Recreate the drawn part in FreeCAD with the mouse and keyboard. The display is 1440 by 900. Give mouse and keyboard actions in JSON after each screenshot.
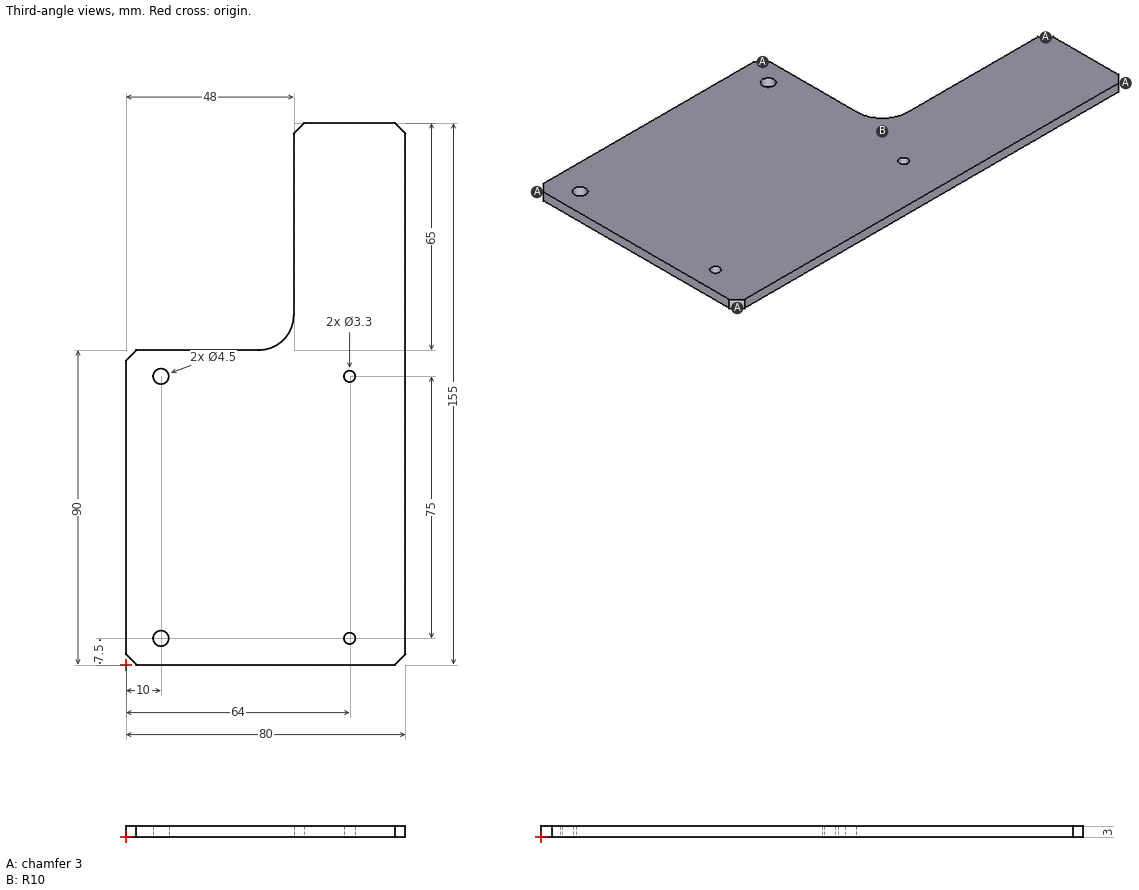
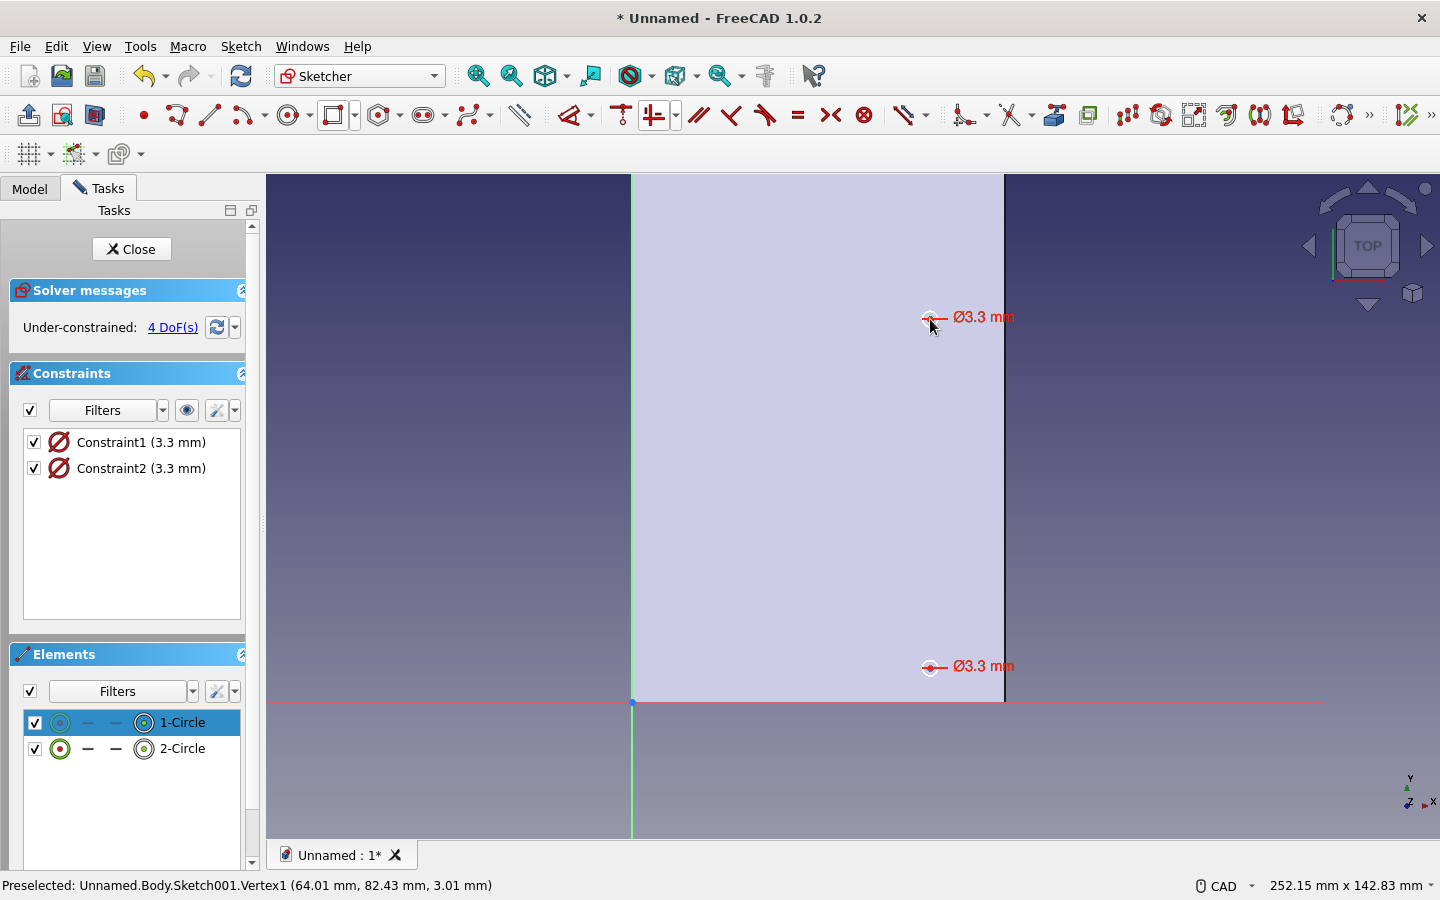
{"action": "left_click", "coordinate": [930, 668]}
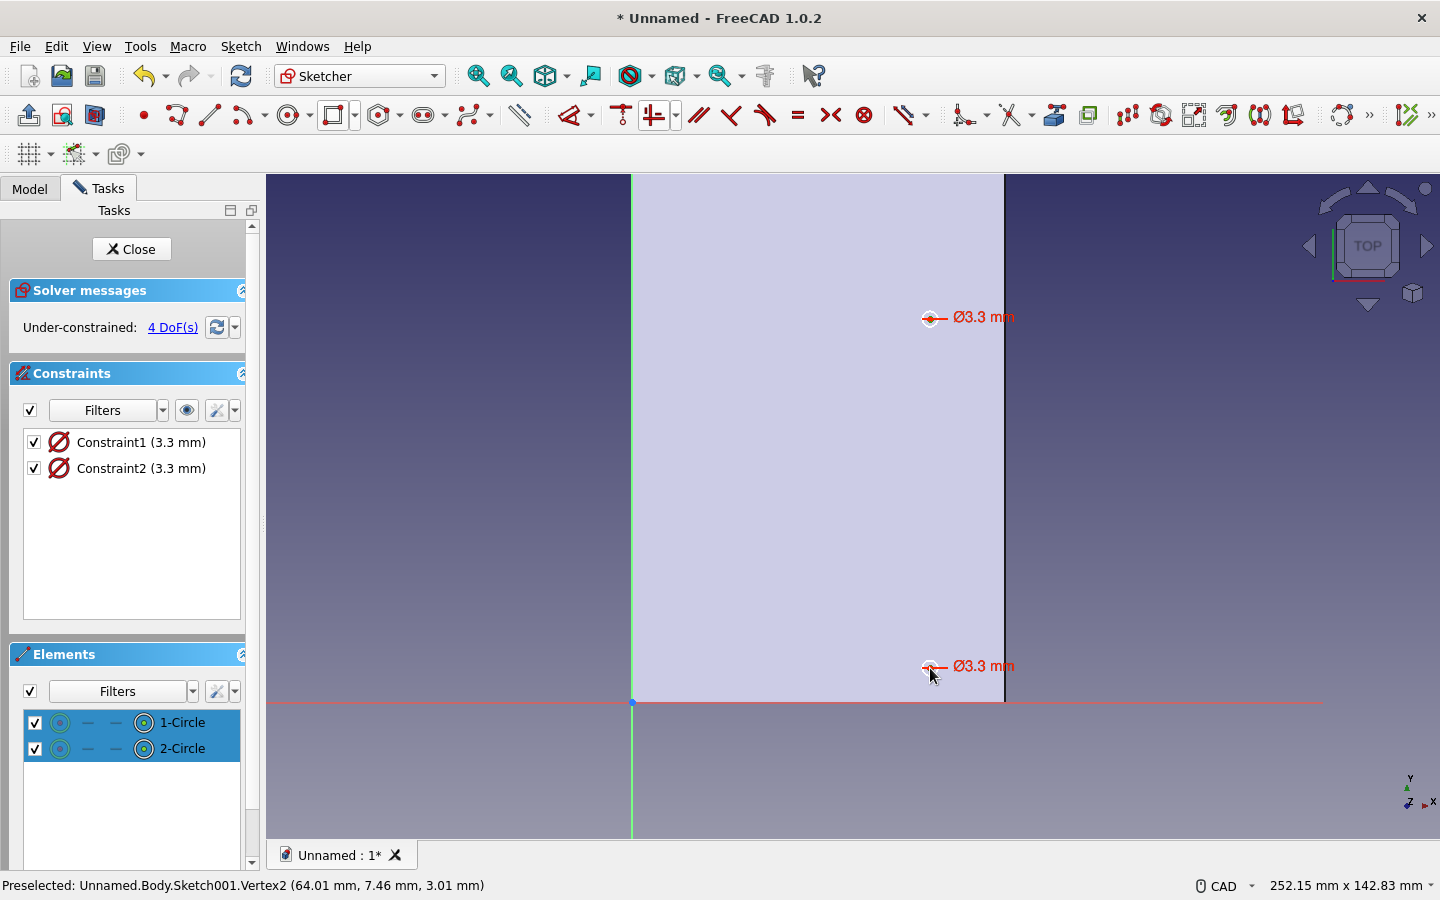
{"action": "key", "text": "v"}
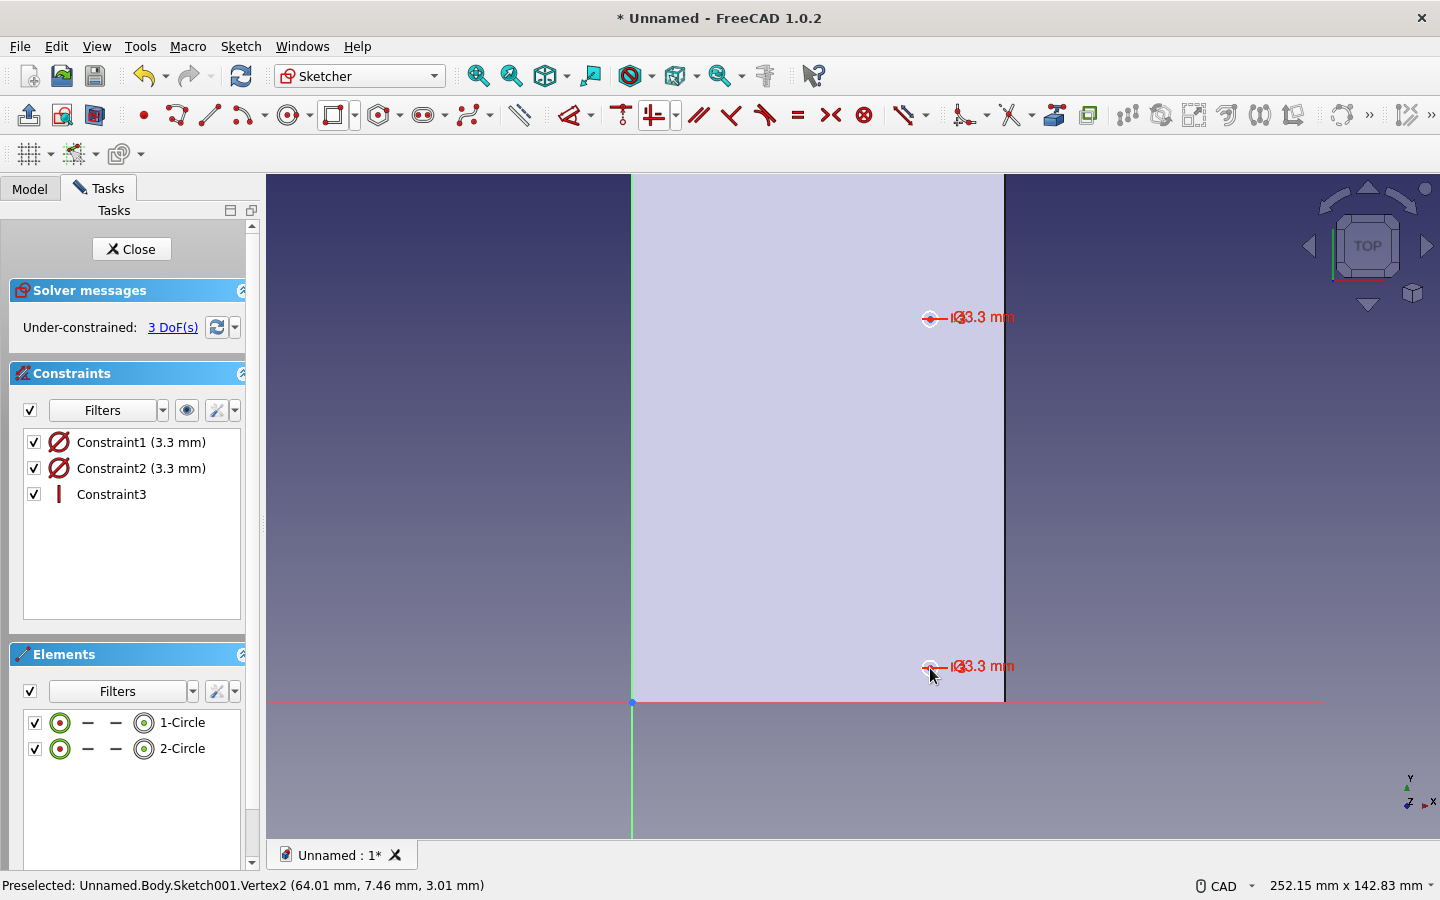
{"action": "key", "text": "d"}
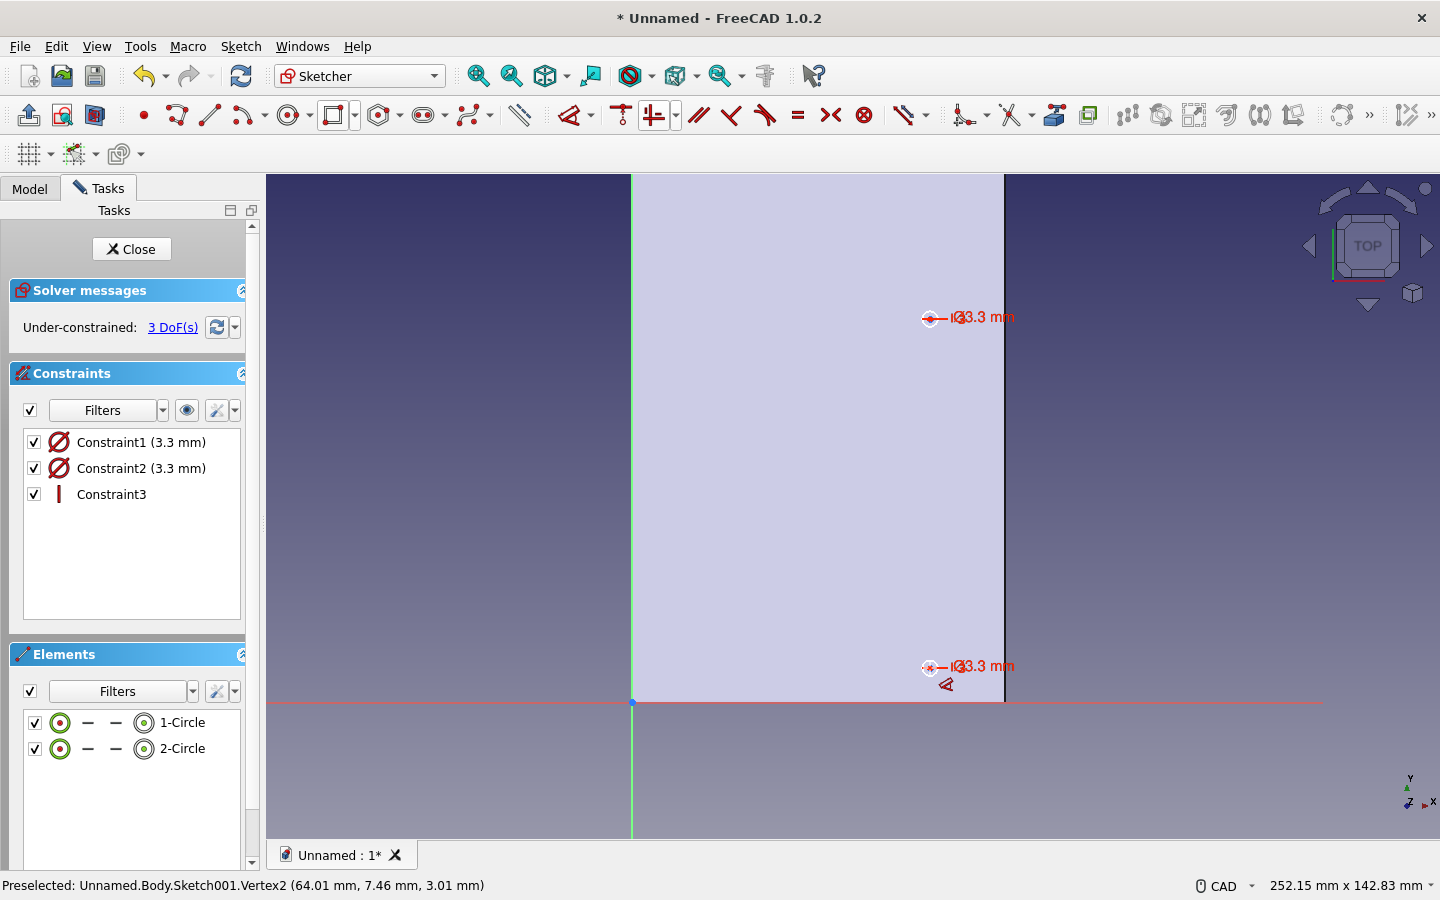
{"action": "left_click", "coordinate": [930, 319]}
{"action": "left_click", "coordinate": [781, 737]}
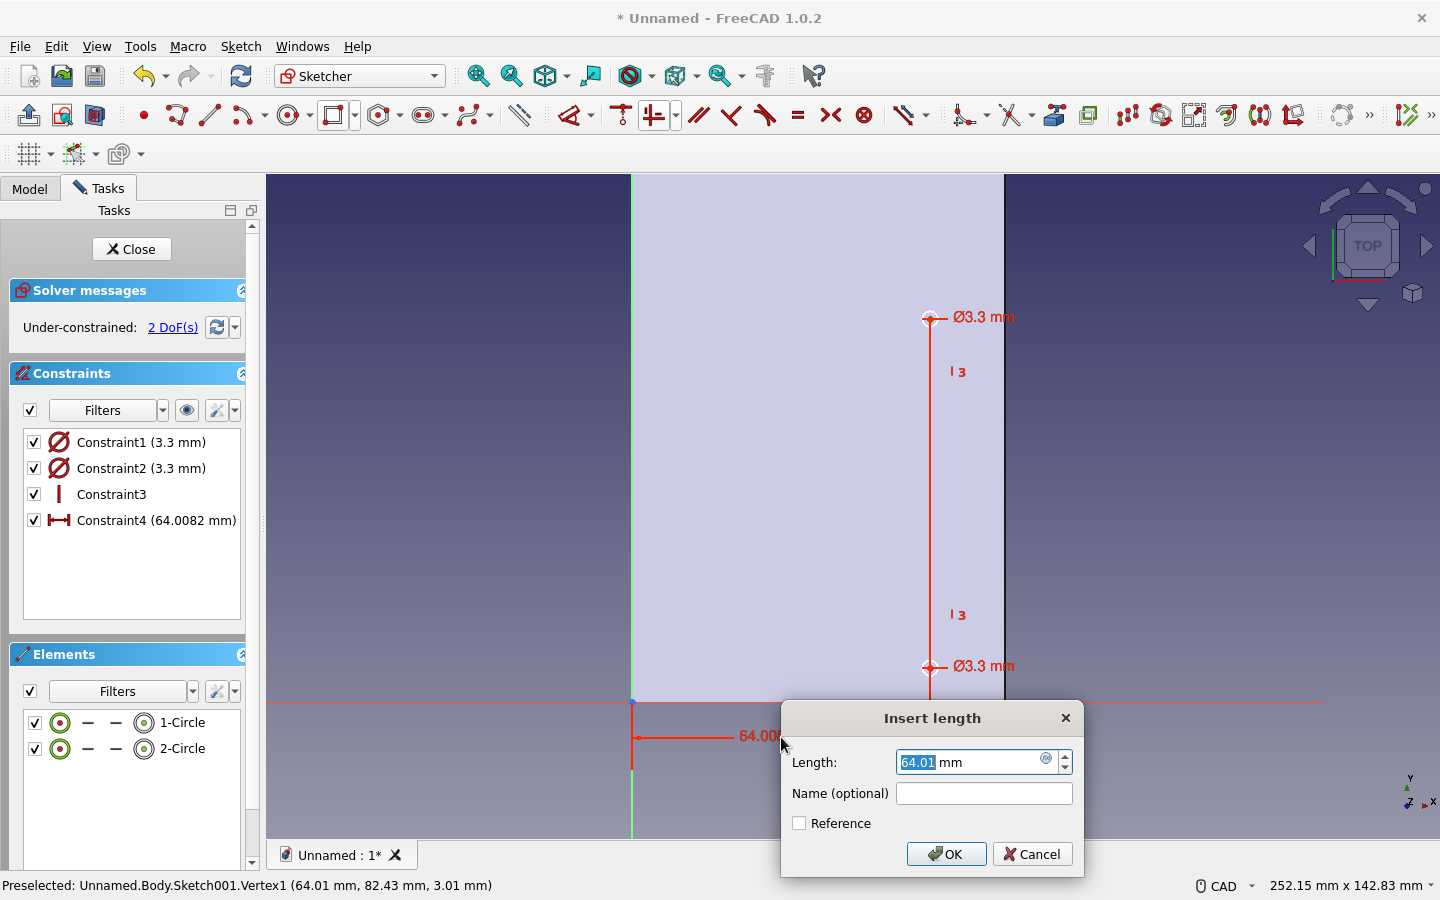
{"action": "type", "text": "64"}
{"action": "key", "text": "Return"}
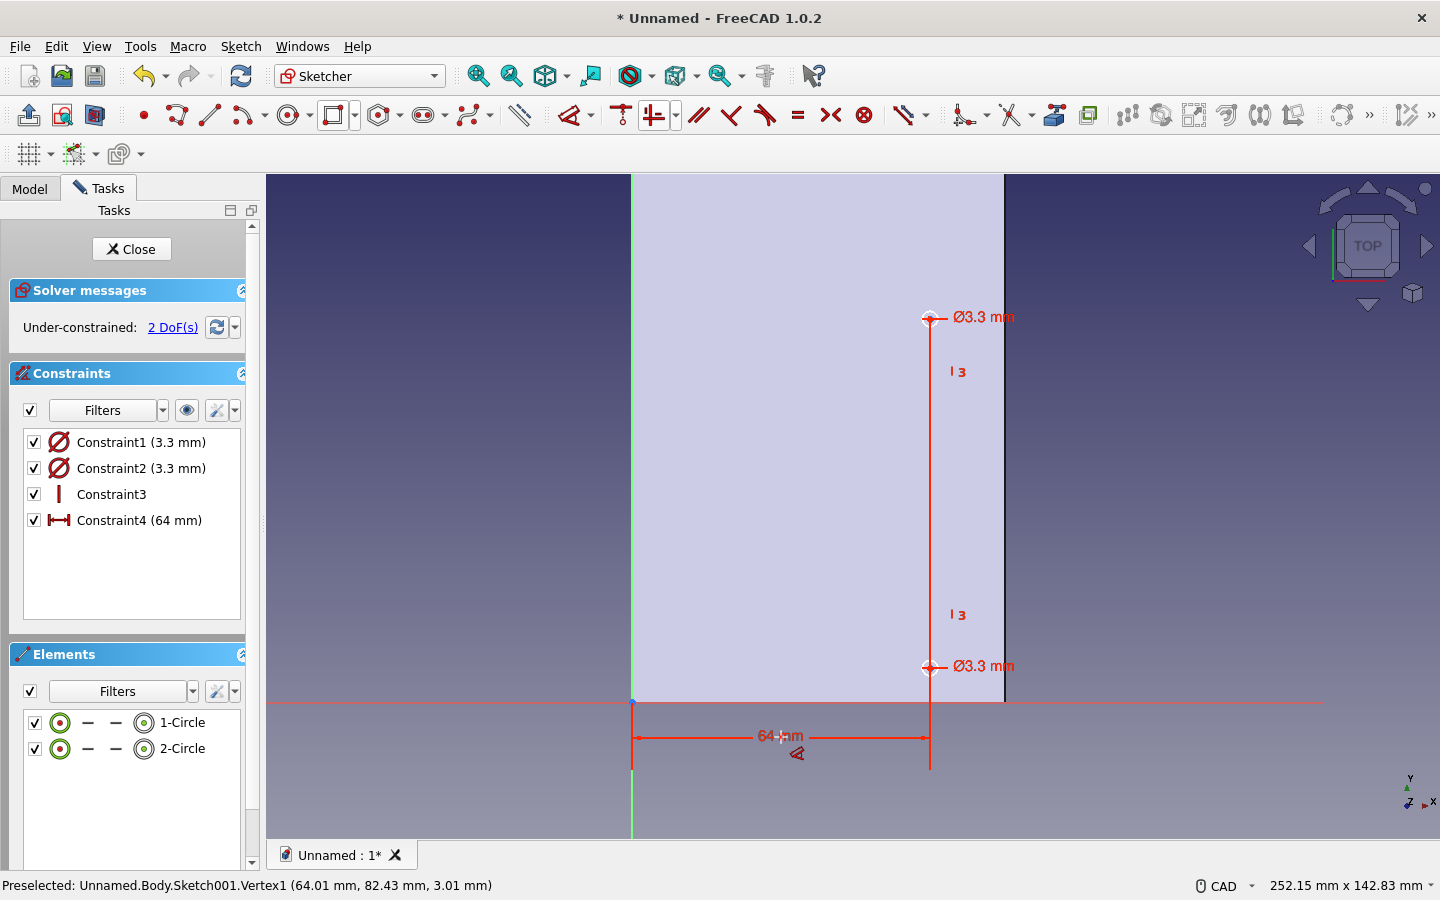
{"action": "left_click", "coordinate": [930, 668]}
{"action": "left_click", "coordinate": [598, 686]}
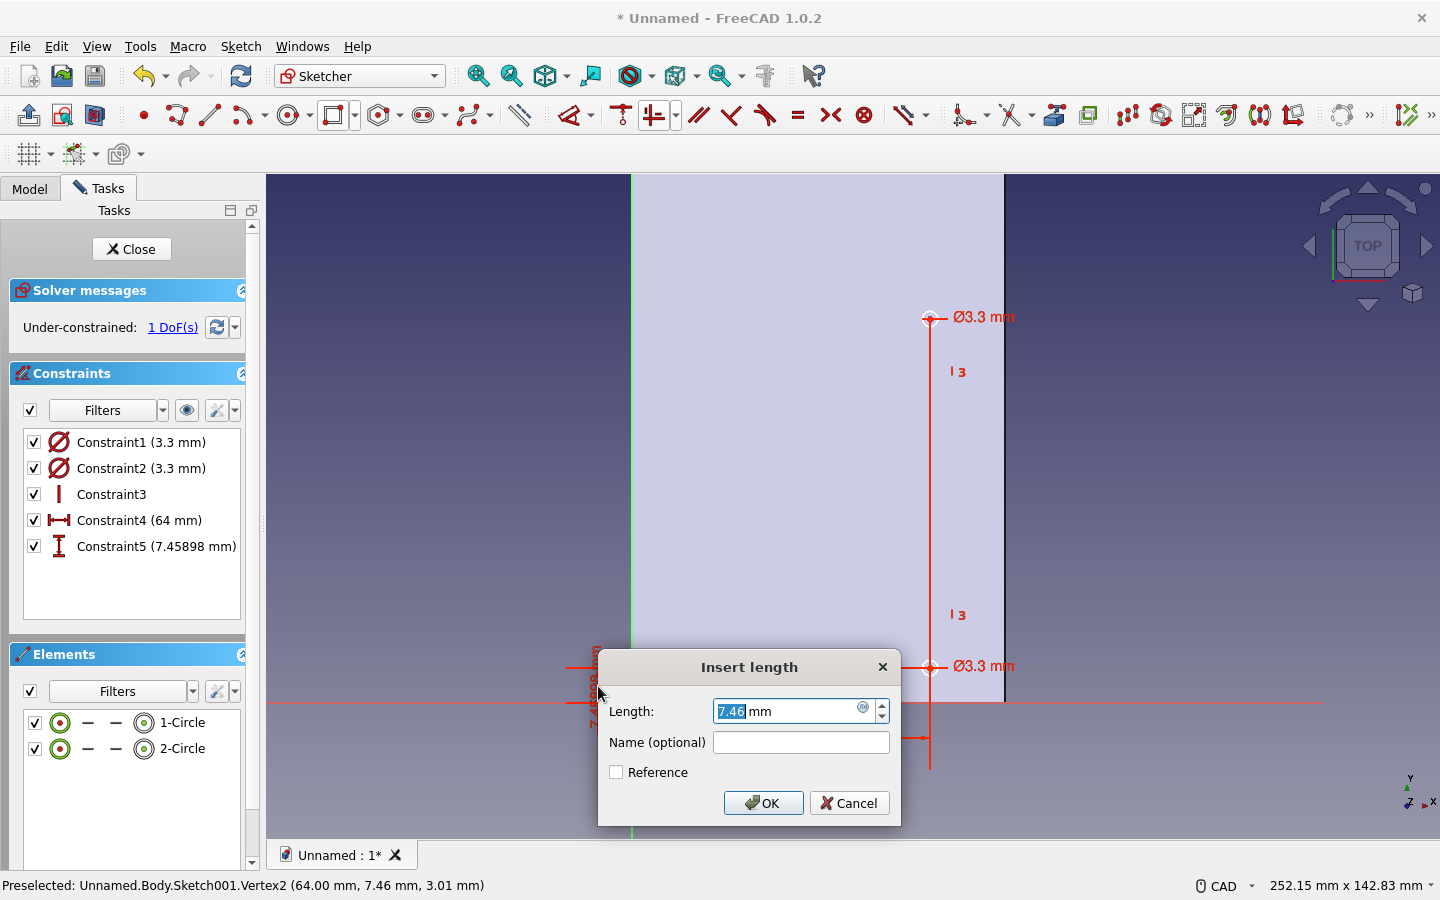
{"action": "type", "text": "7.5"}
{"action": "key", "text": "Return"}